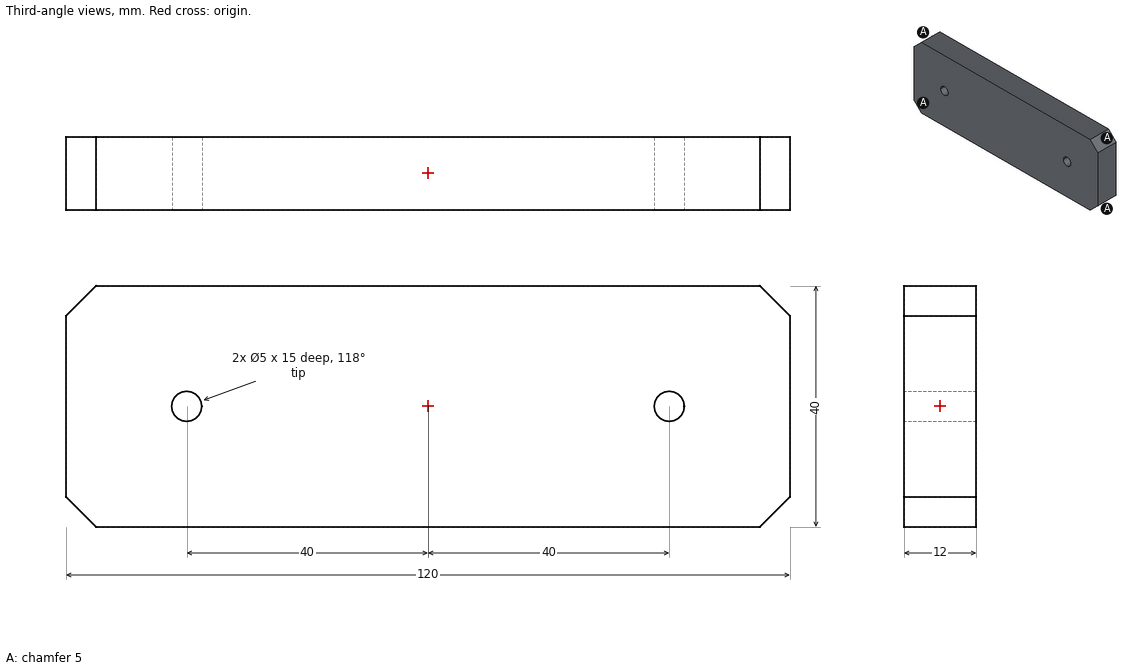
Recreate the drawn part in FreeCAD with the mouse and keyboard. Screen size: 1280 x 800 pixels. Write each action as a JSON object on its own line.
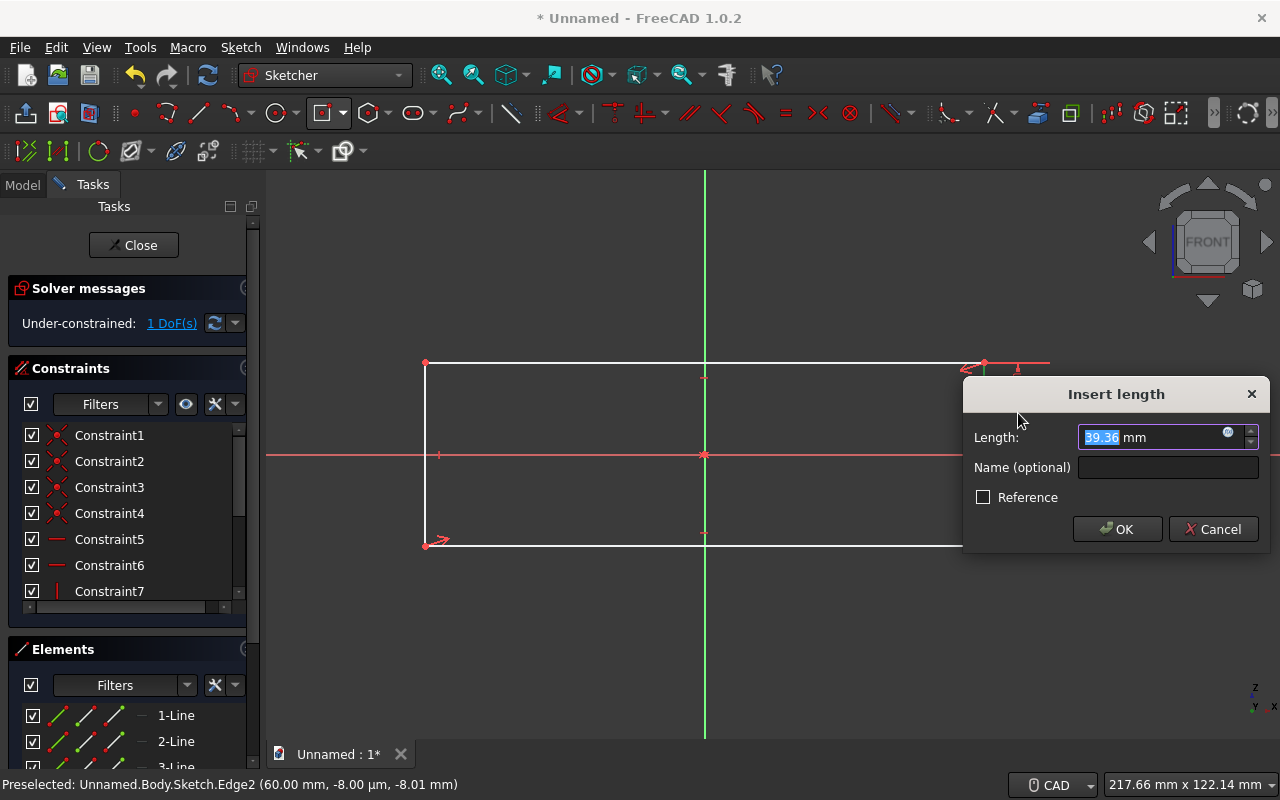
{"action": "type", "text": "40"}
{"action": "key", "text": "Return"}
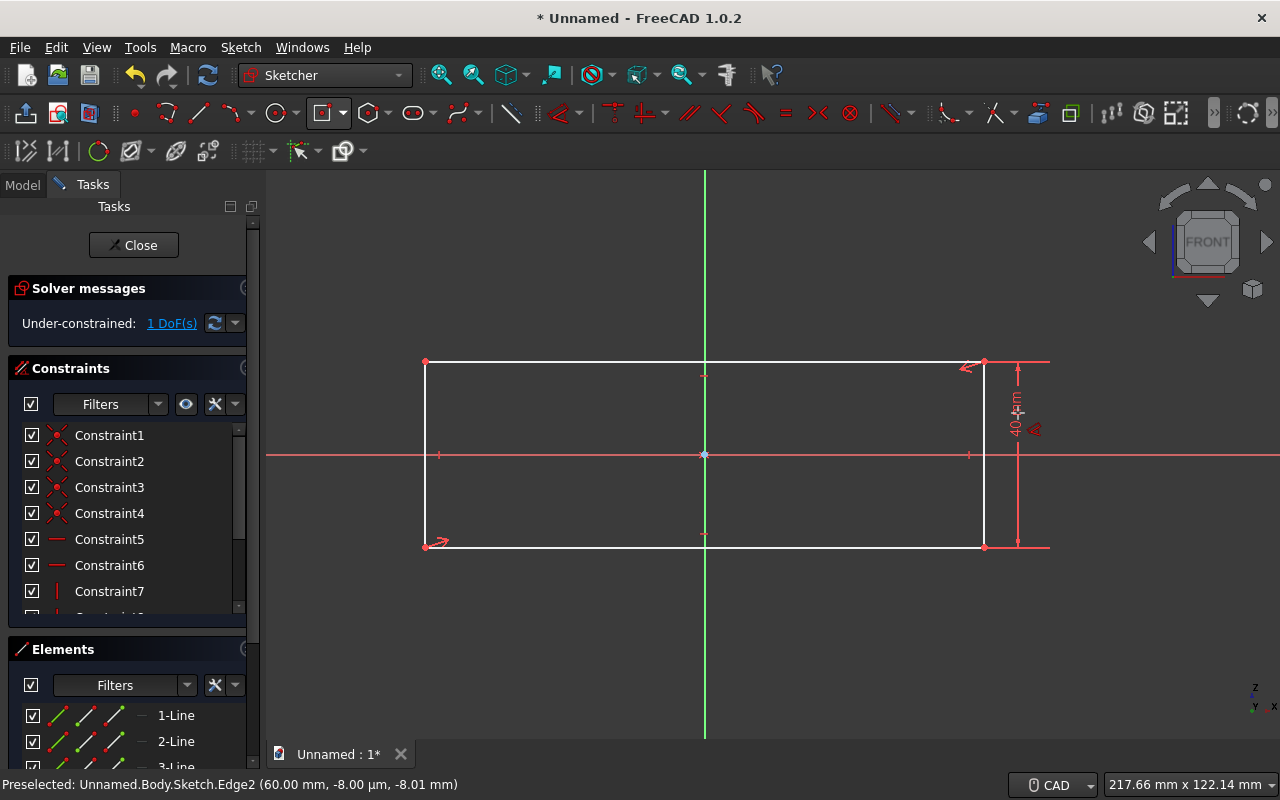
{"action": "left_click", "coordinate": [593, 548]}
{"action": "left_click", "coordinate": [576, 582]}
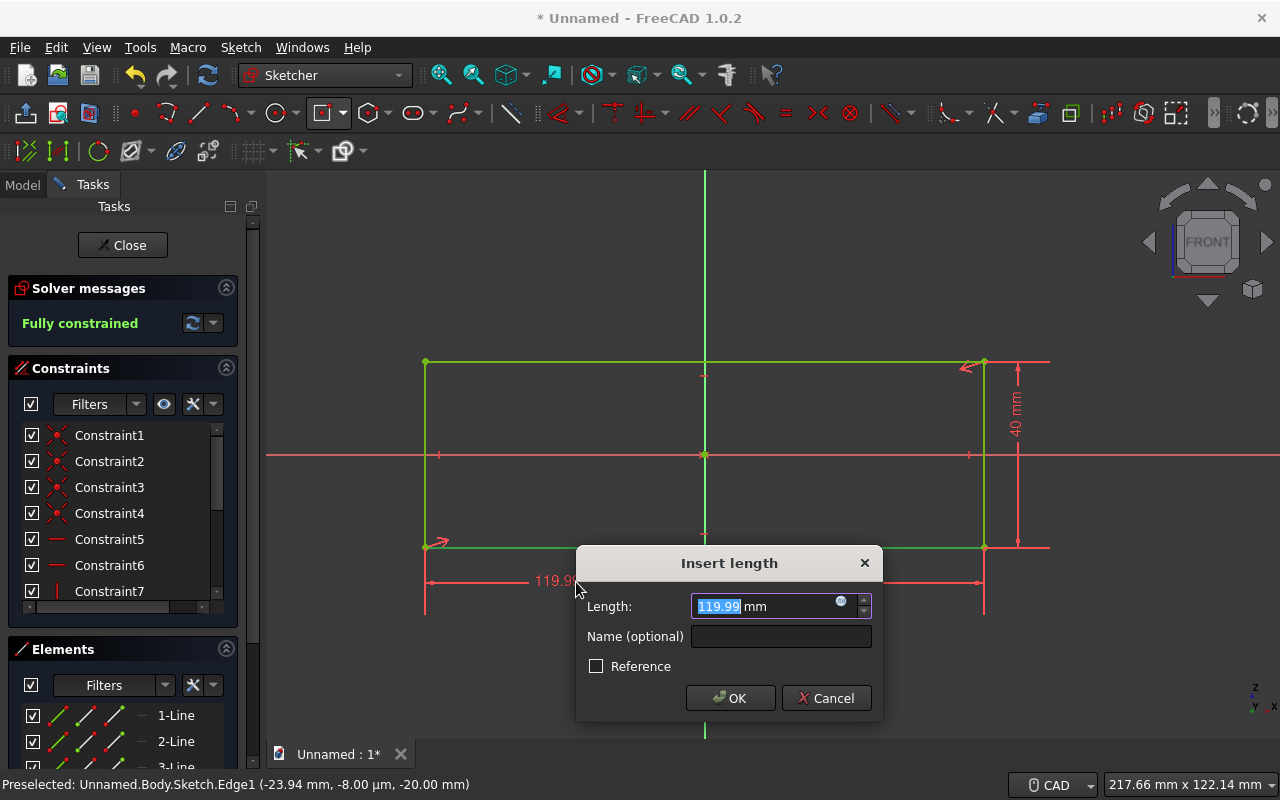
{"action": "type", "text": "120"}
{"action": "key", "text": "Return"}
{"action": "key", "text": "Escape"}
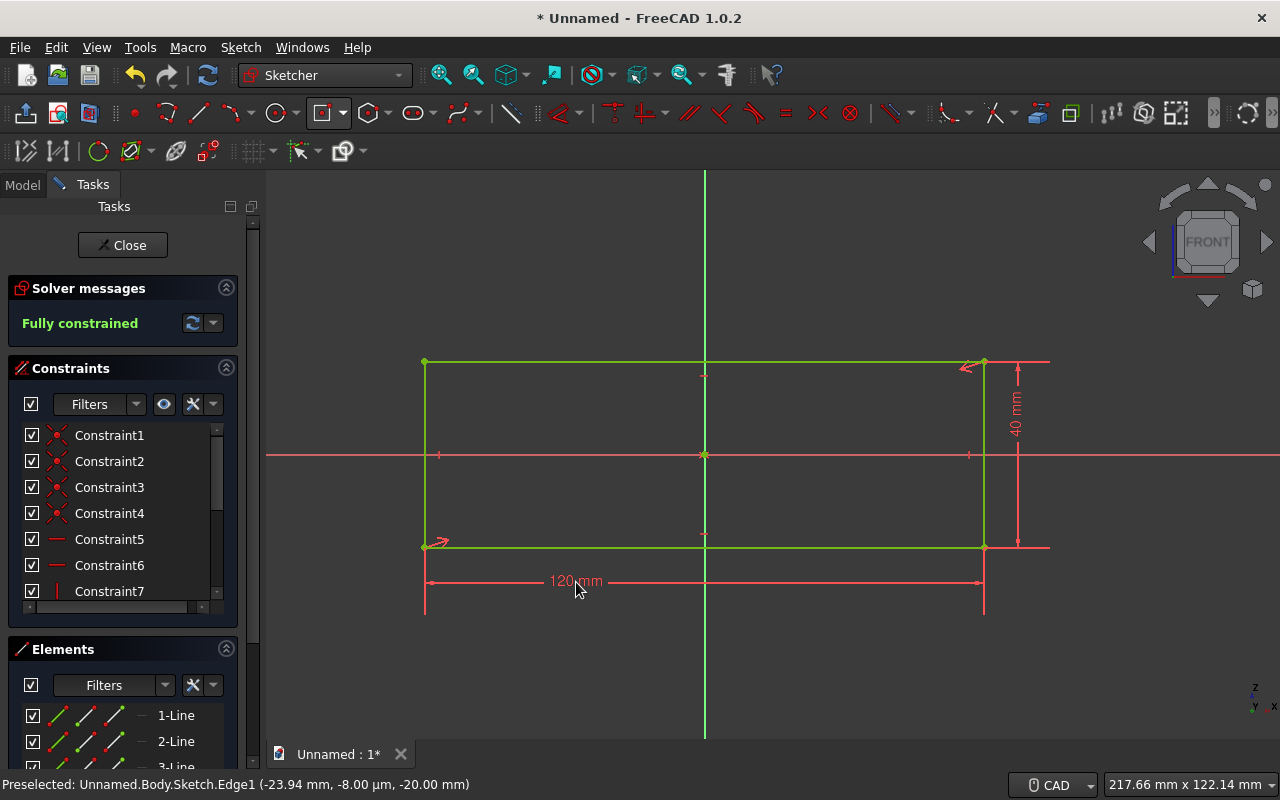
{"action": "left_click", "coordinate": [123, 245]}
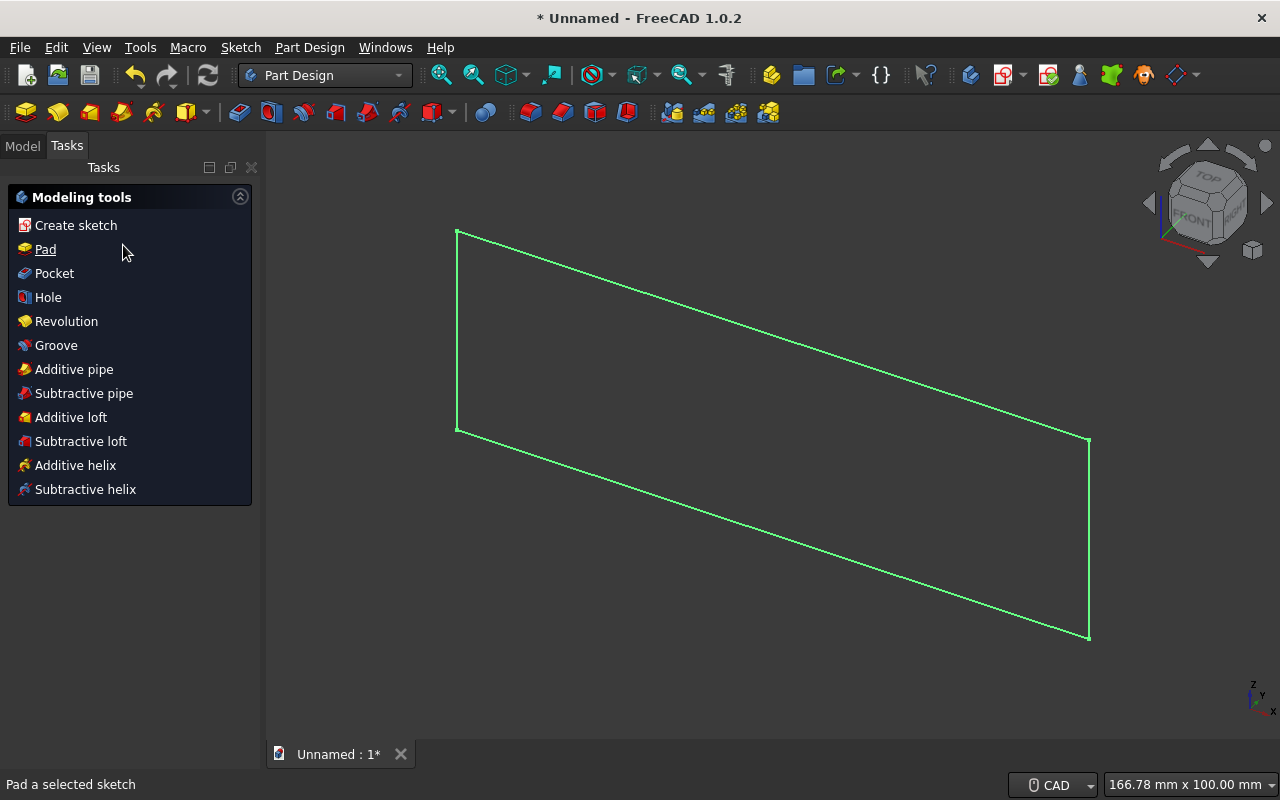
{"action": "left_click", "coordinate": [26, 112]}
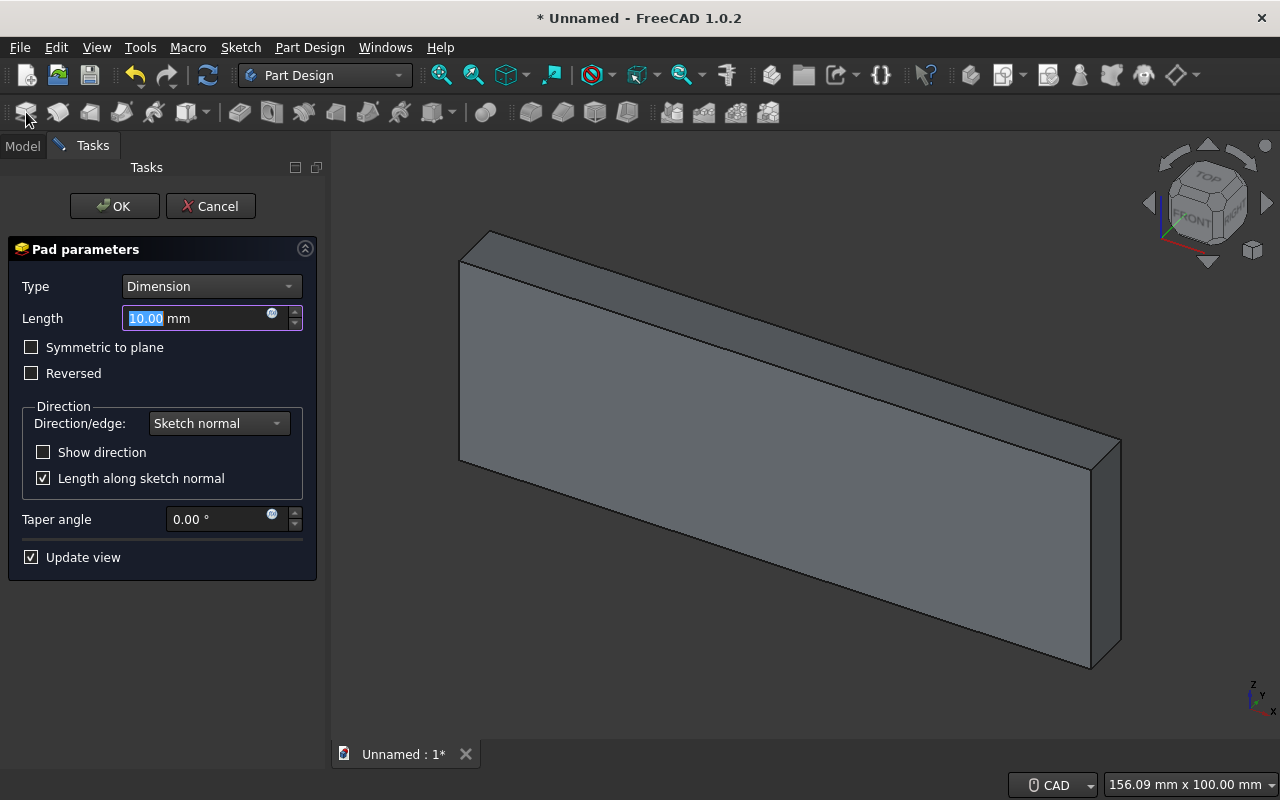
{"action": "type", "text": "12"}
{"action": "key", "text": "Tab"}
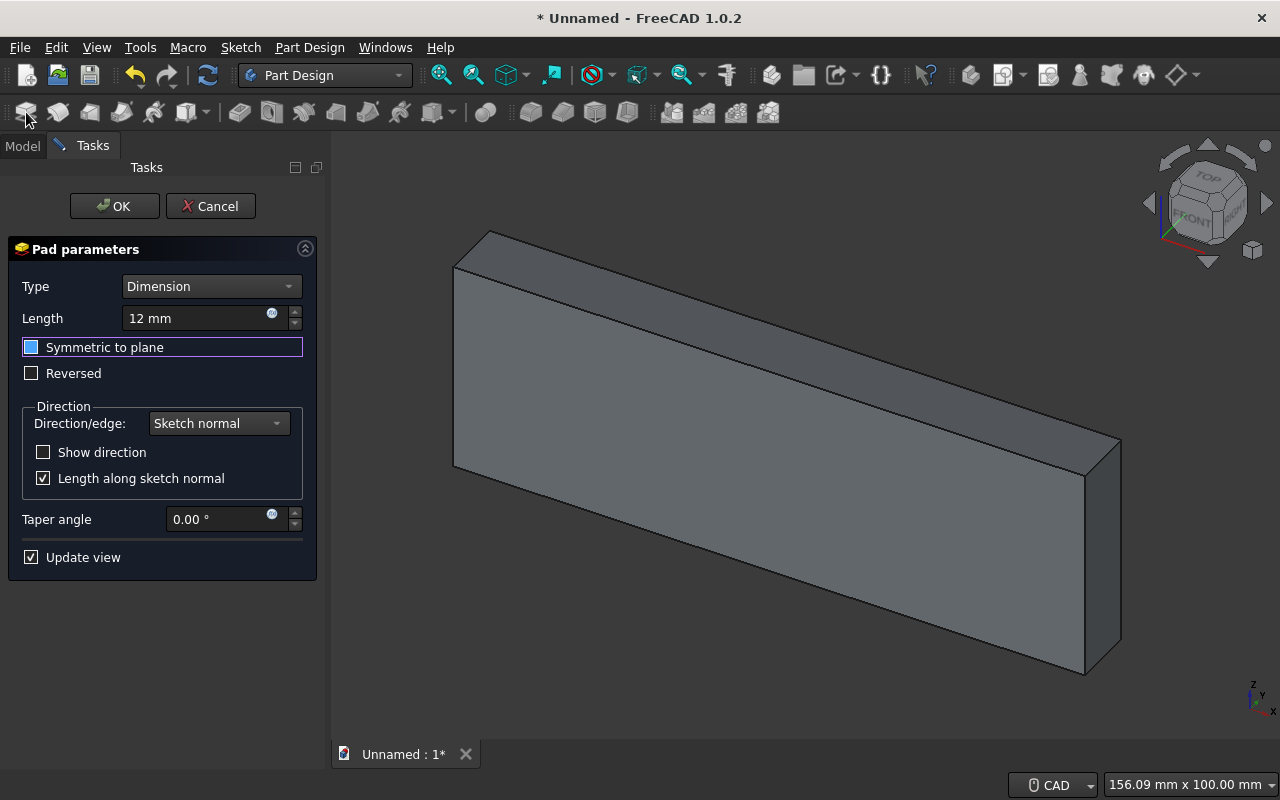
{"action": "left_click", "coordinate": [30, 347]}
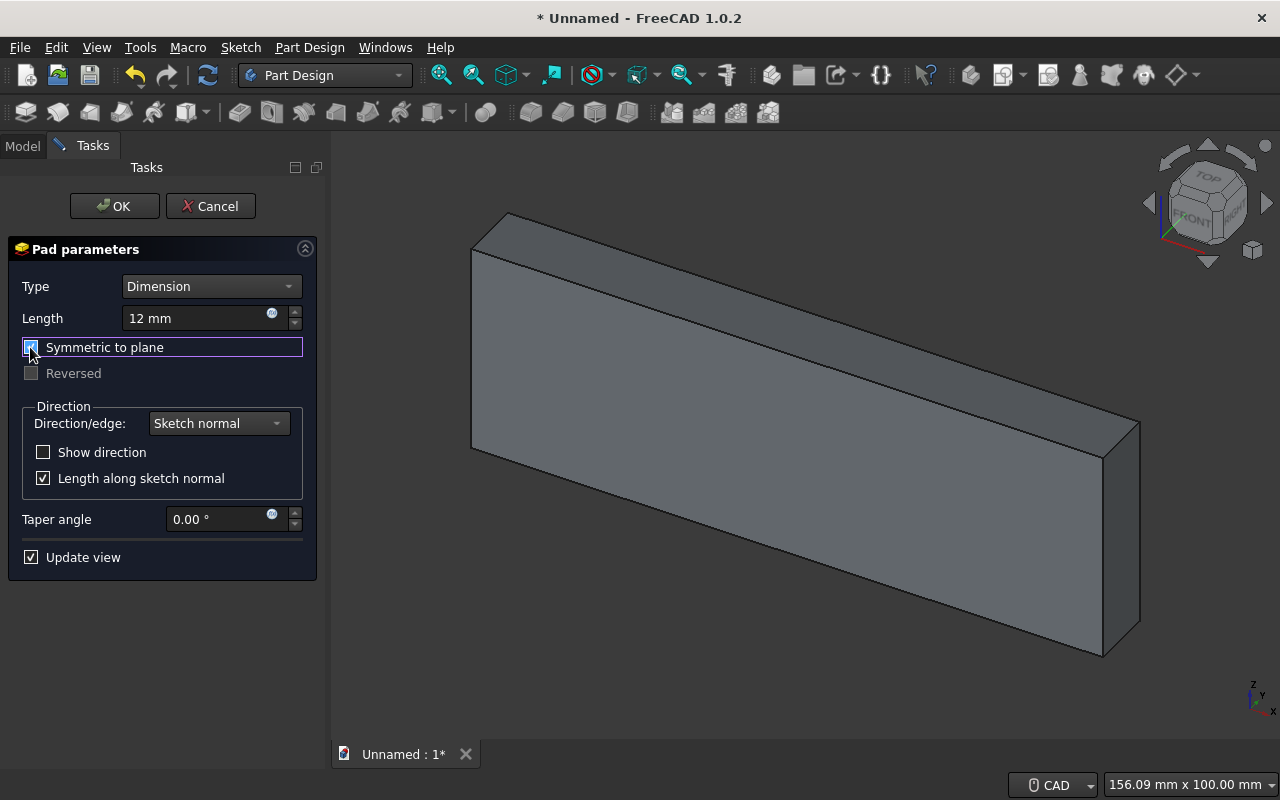
{"action": "left_click", "coordinate": [115, 206]}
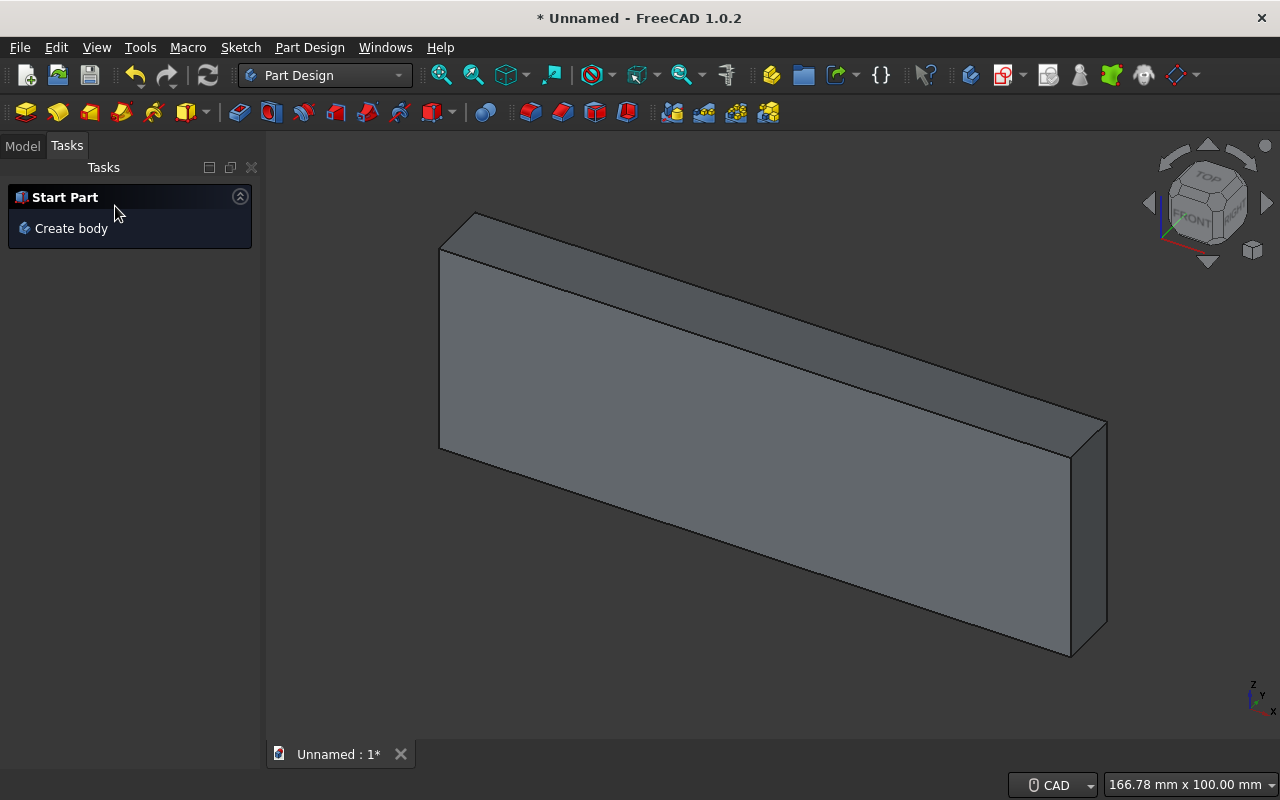
{"action": "key", "text": "4"}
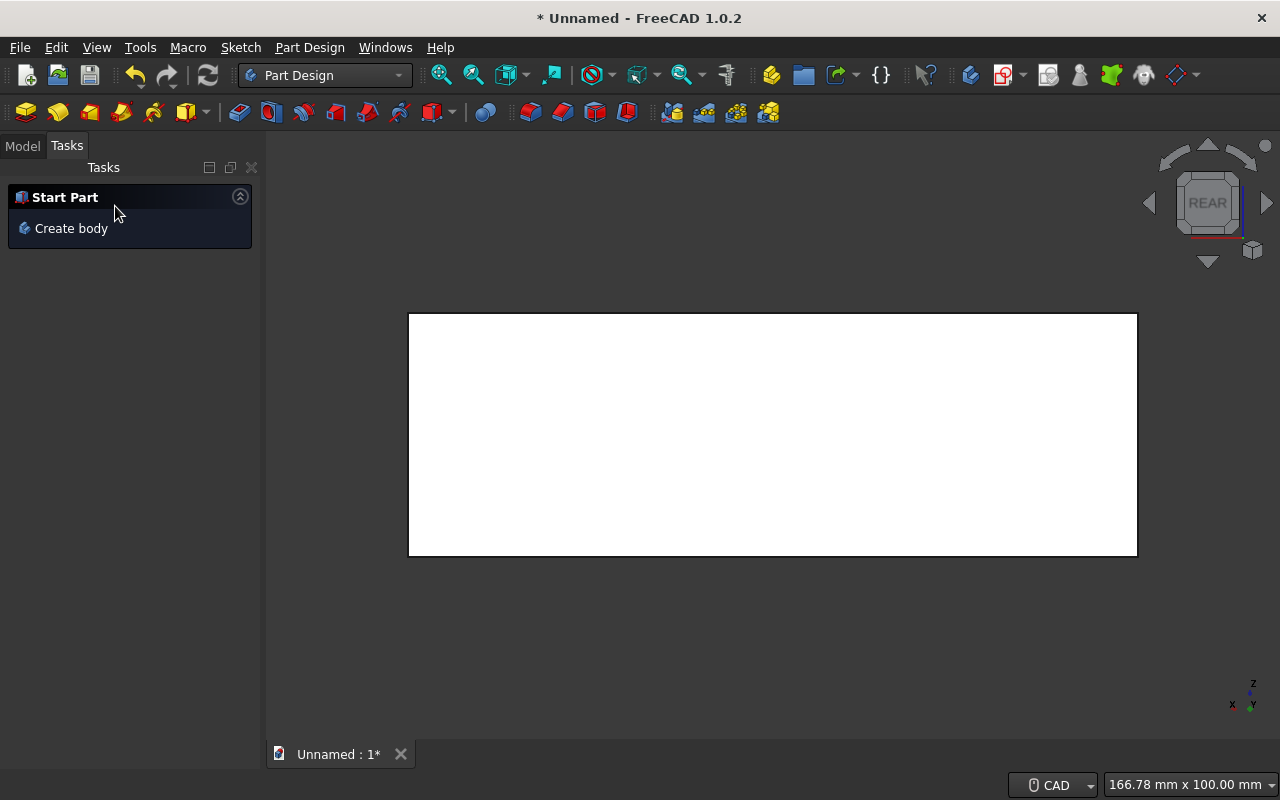
{"action": "left_click", "coordinate": [565, 434]}